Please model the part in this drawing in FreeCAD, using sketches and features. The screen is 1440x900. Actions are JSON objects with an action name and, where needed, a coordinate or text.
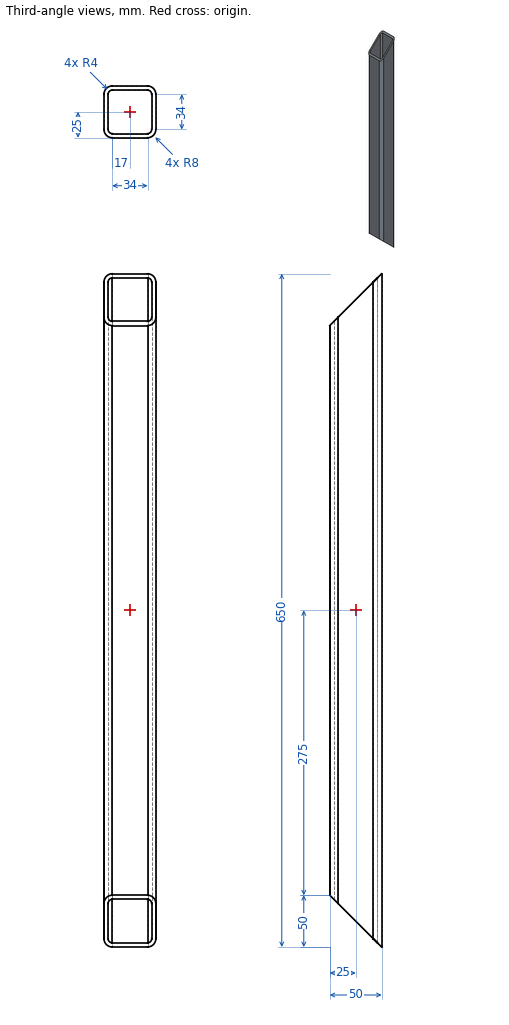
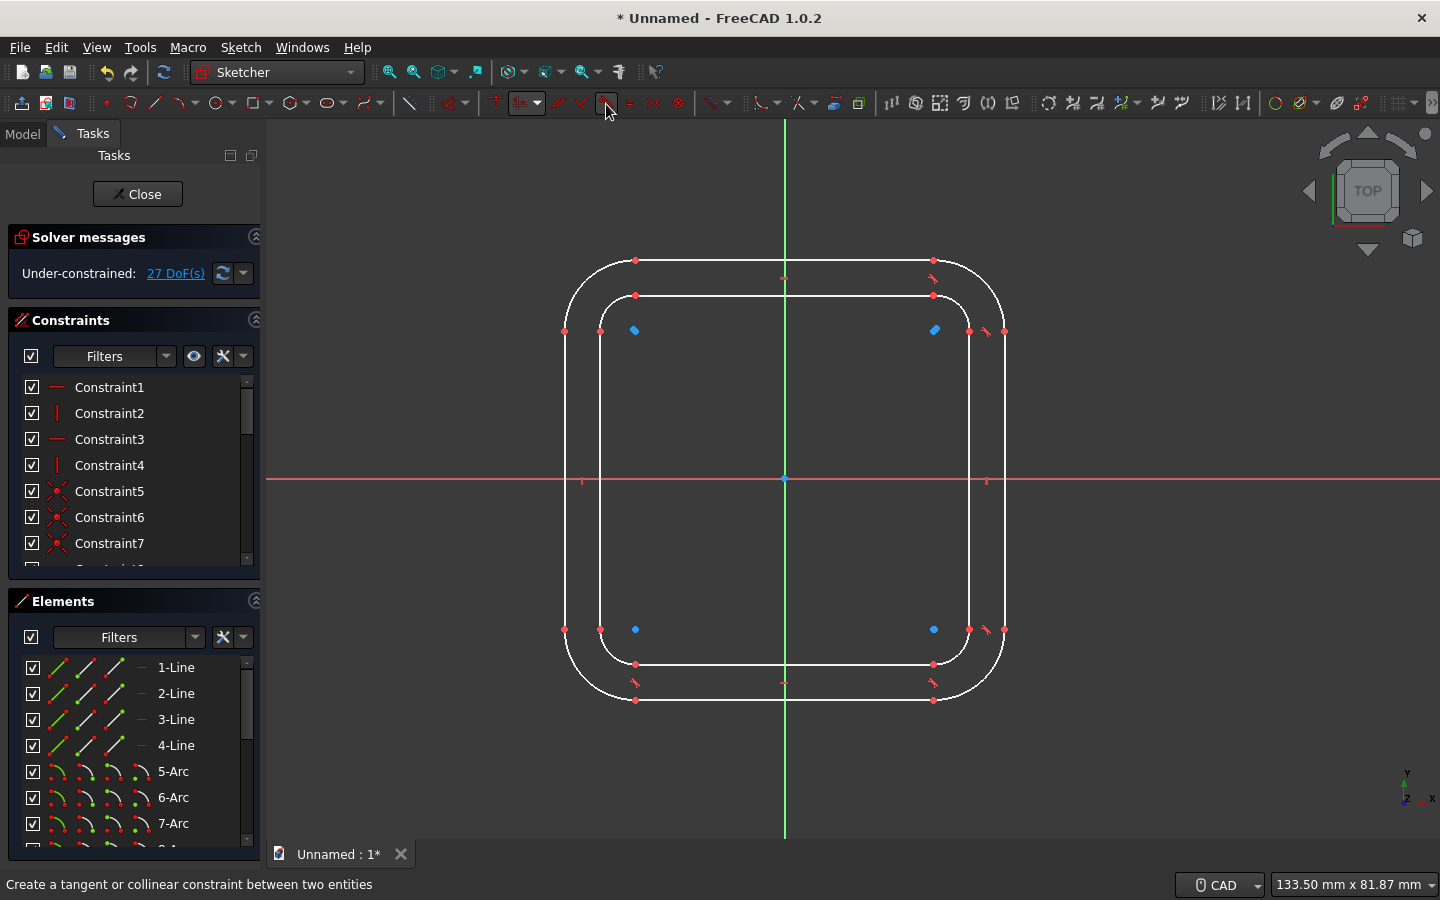
{"action": "left_click", "coordinate": [844, 260]}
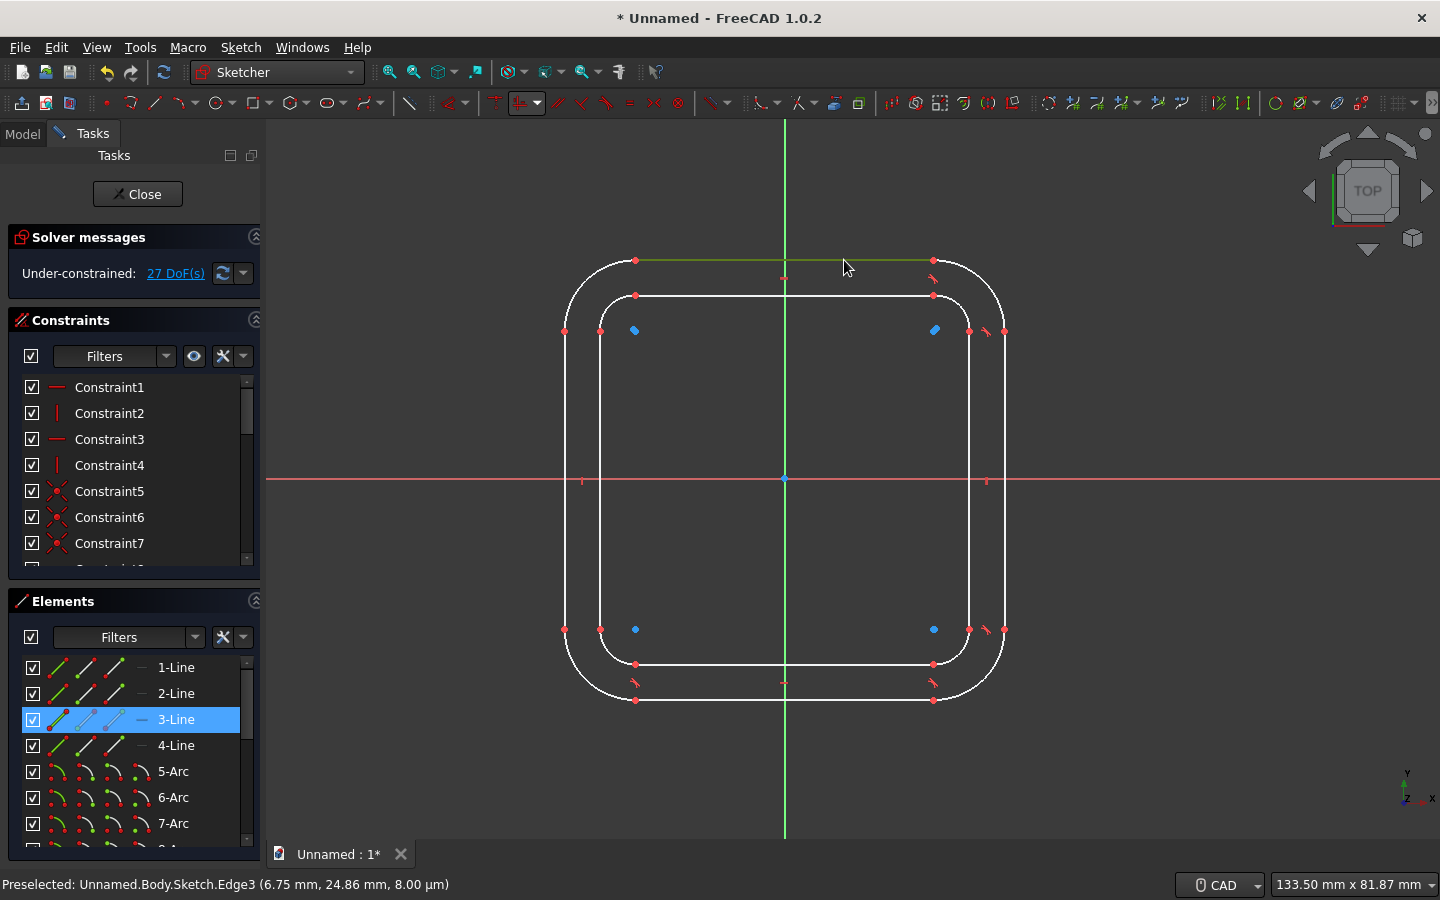
{"action": "left_click", "coordinate": [603, 268]}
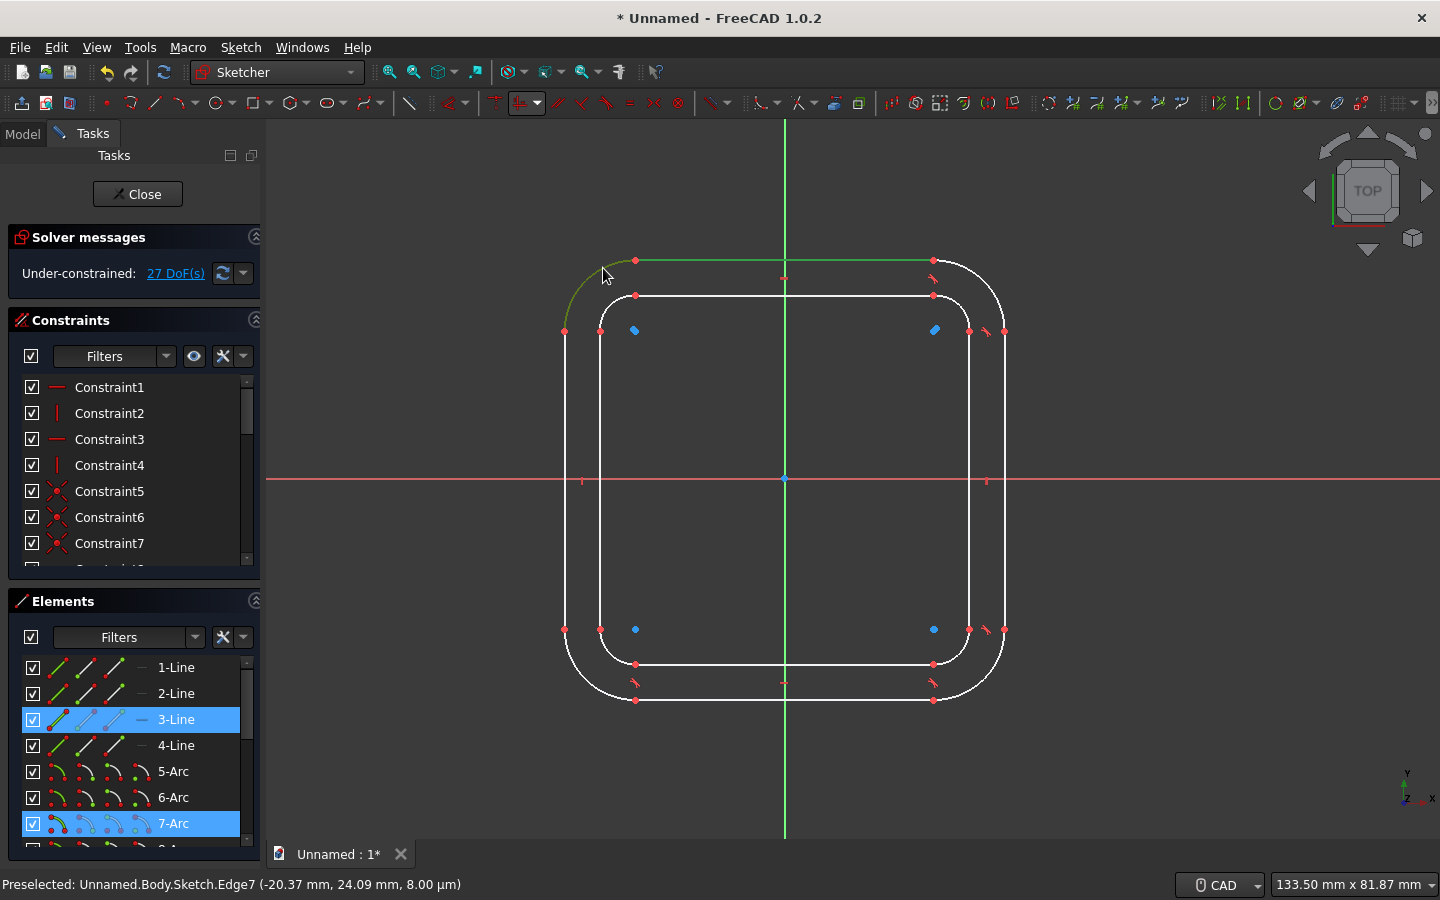
{"action": "left_click", "coordinate": [606, 104]}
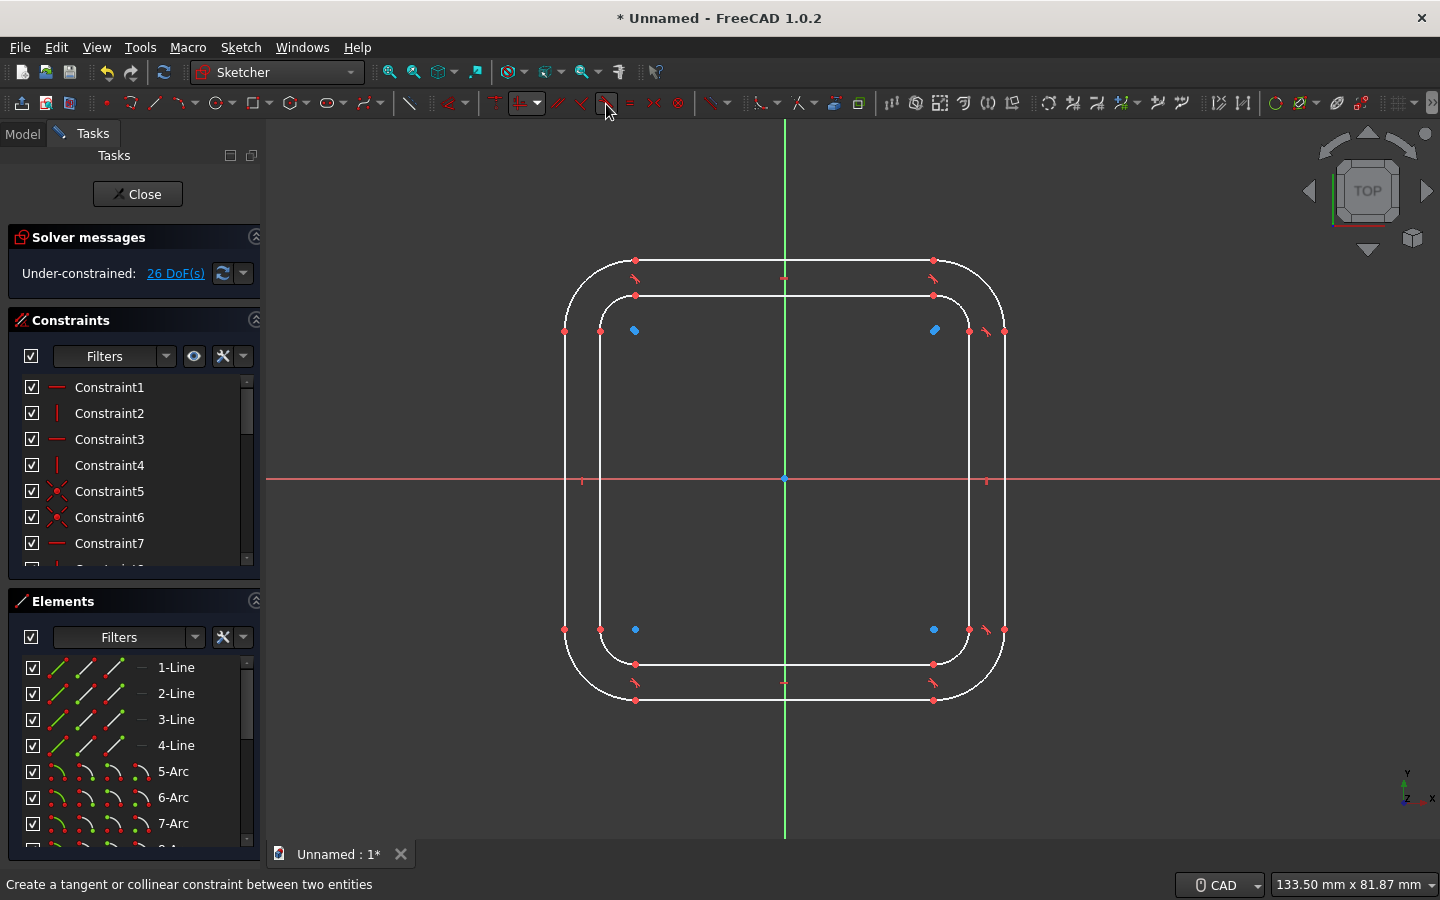
{"action": "left_click", "coordinate": [565, 421]}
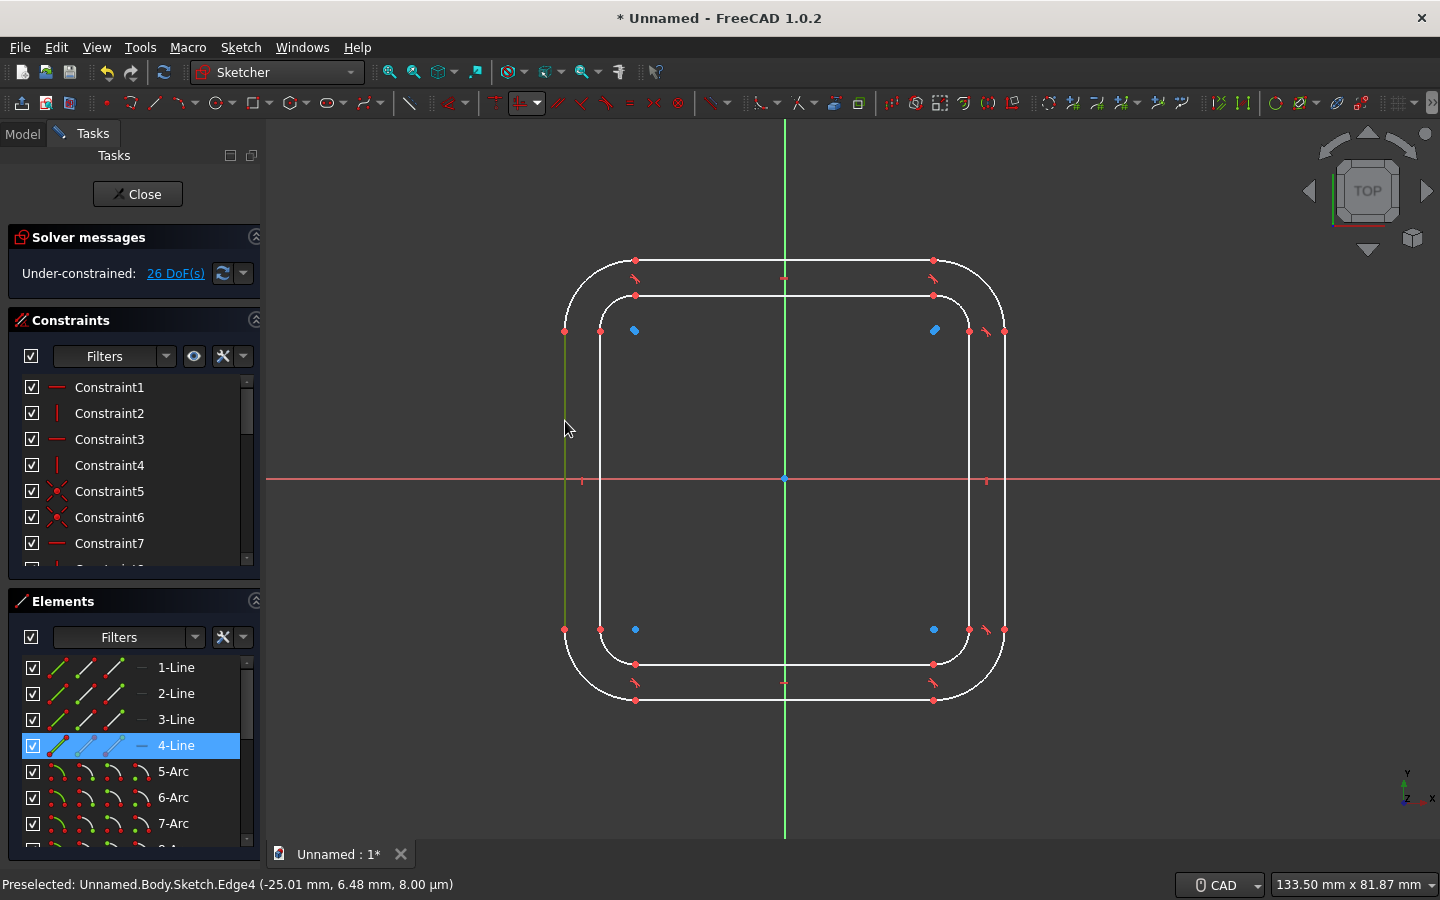
{"action": "left_click", "coordinate": [603, 268]}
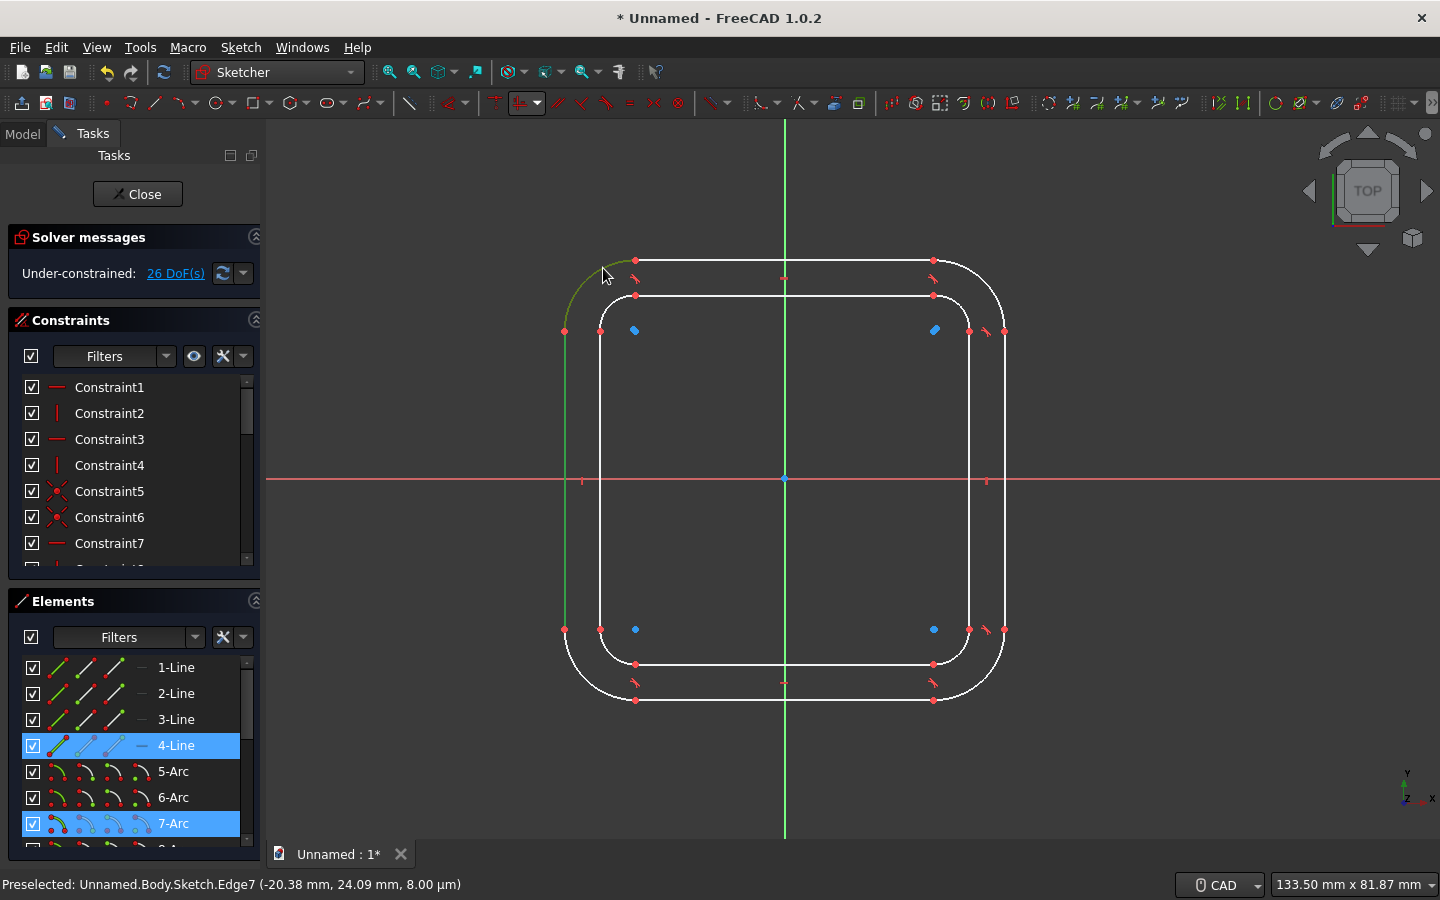
{"action": "left_click", "coordinate": [606, 104]}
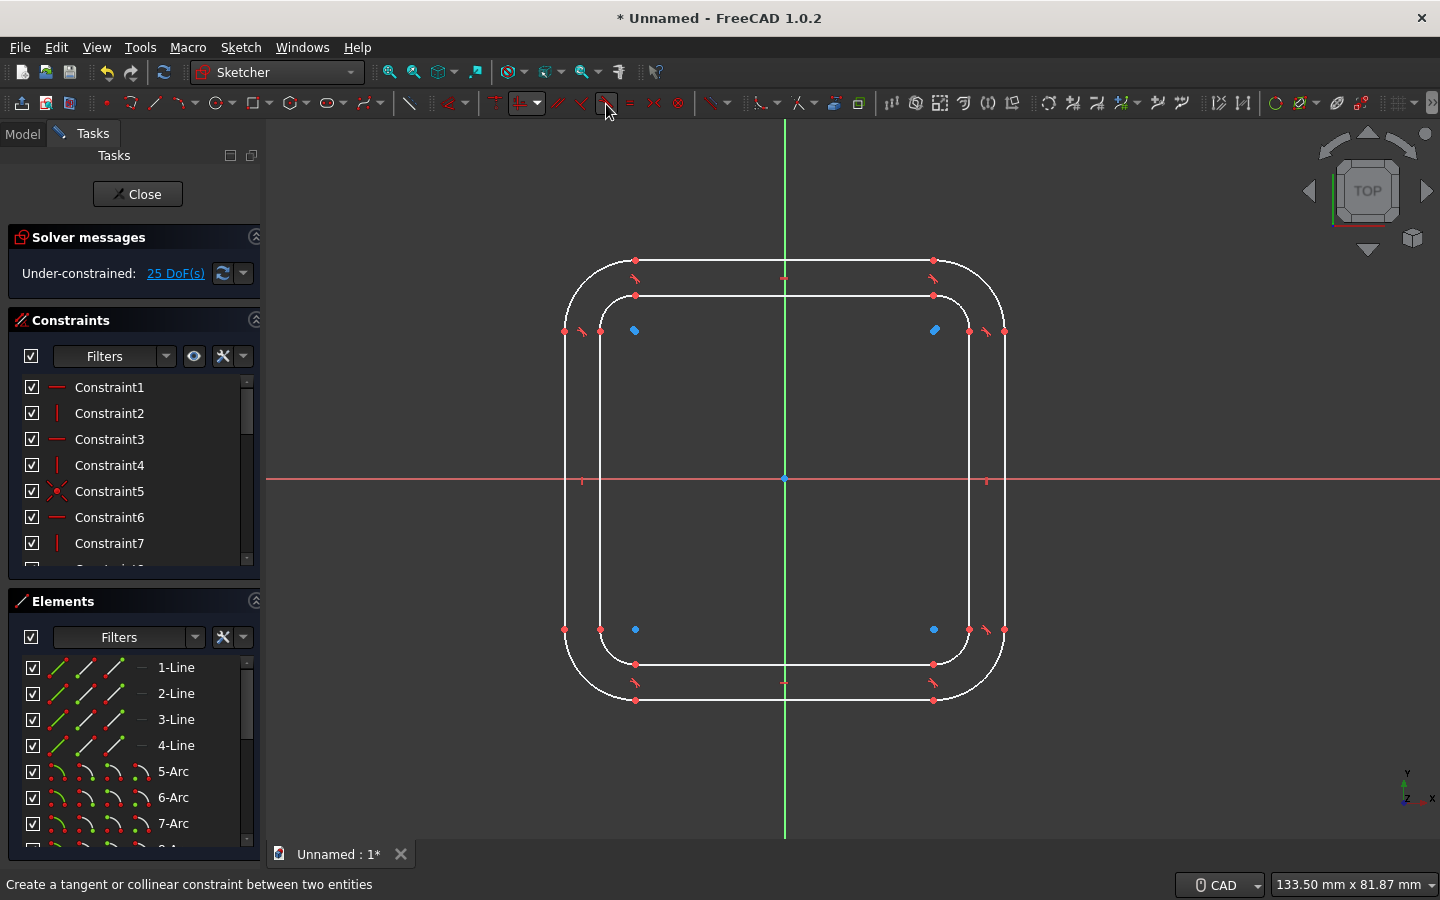
{"action": "left_click", "coordinate": [565, 421]}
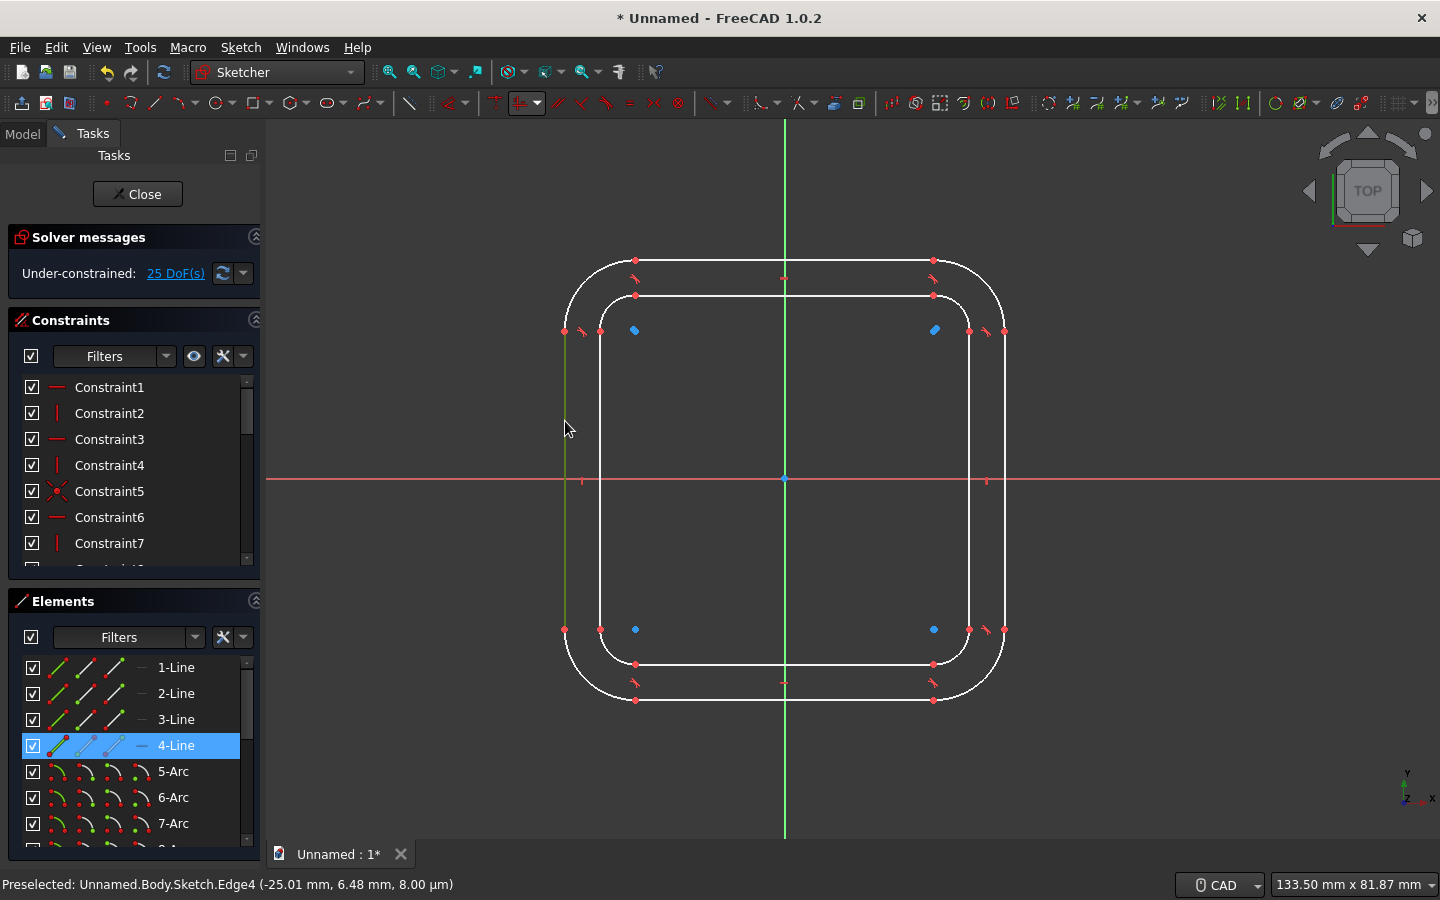
{"action": "left_click", "coordinate": [572, 661]}